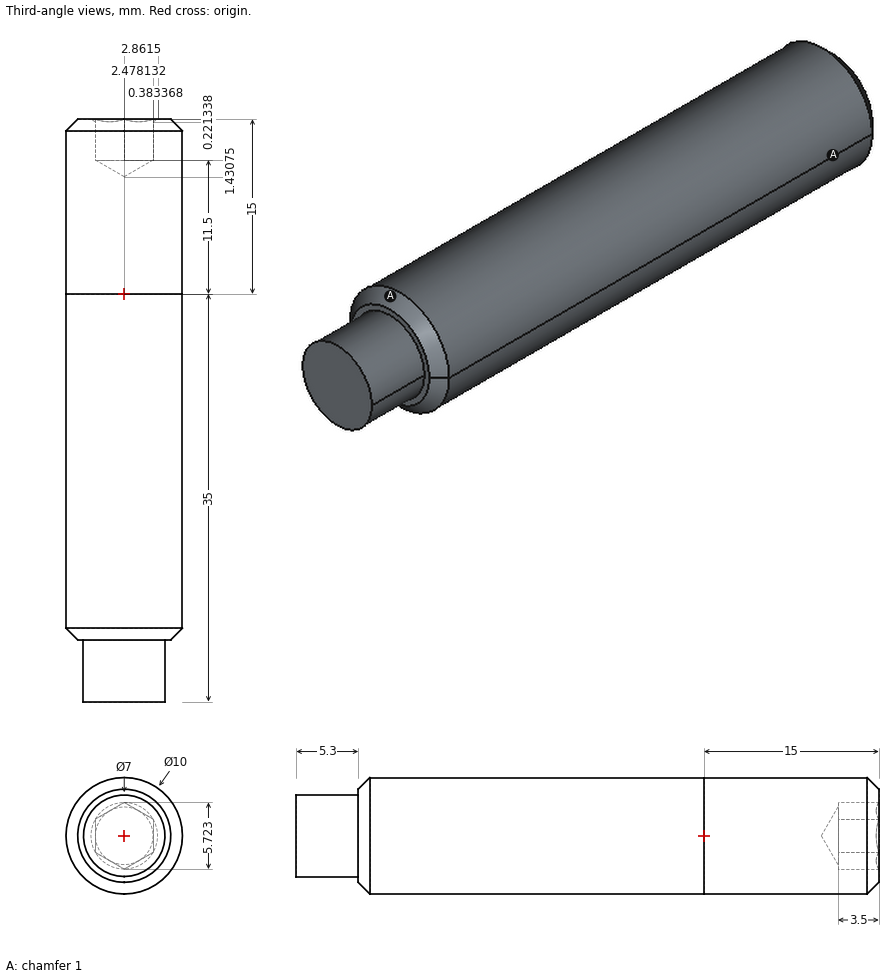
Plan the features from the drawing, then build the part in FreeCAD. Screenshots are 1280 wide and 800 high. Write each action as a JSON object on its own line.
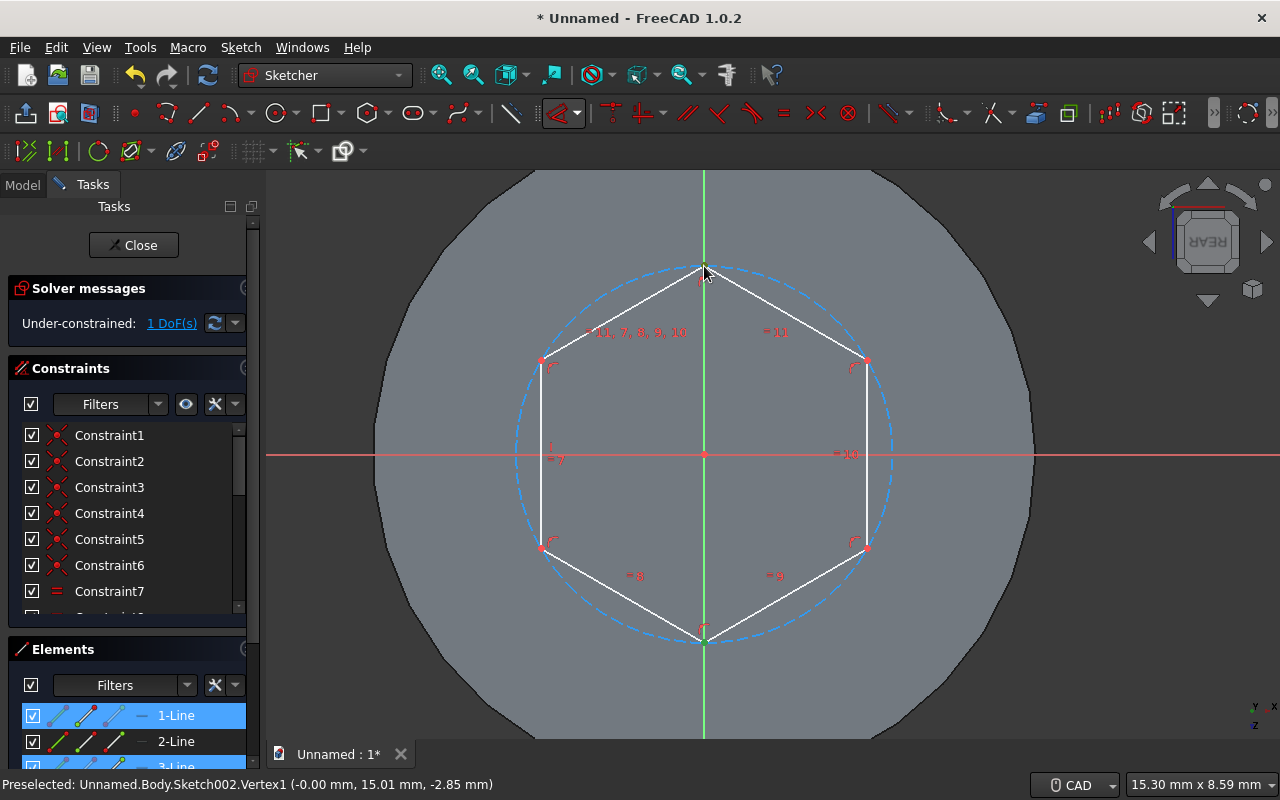
{"action": "left_click", "coordinate": [580, 114]}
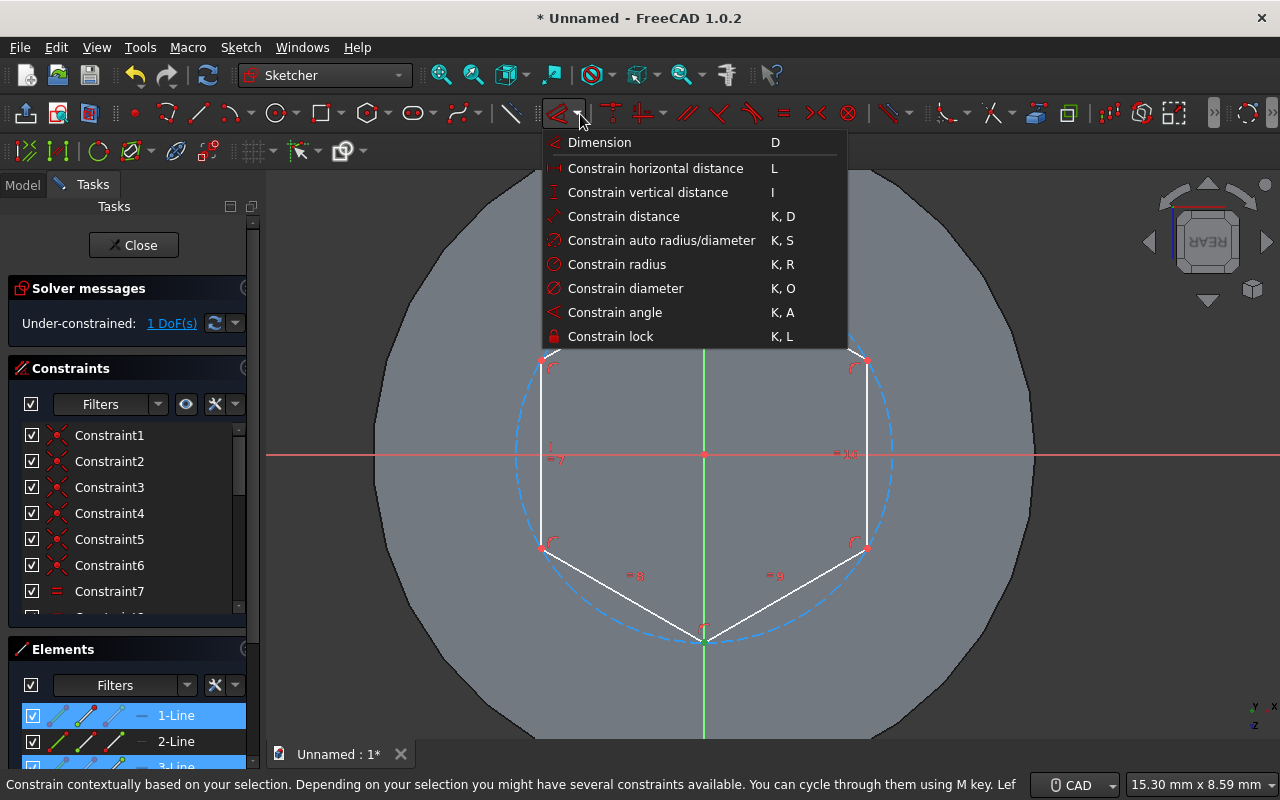
{"action": "left_click", "coordinate": [695, 192]}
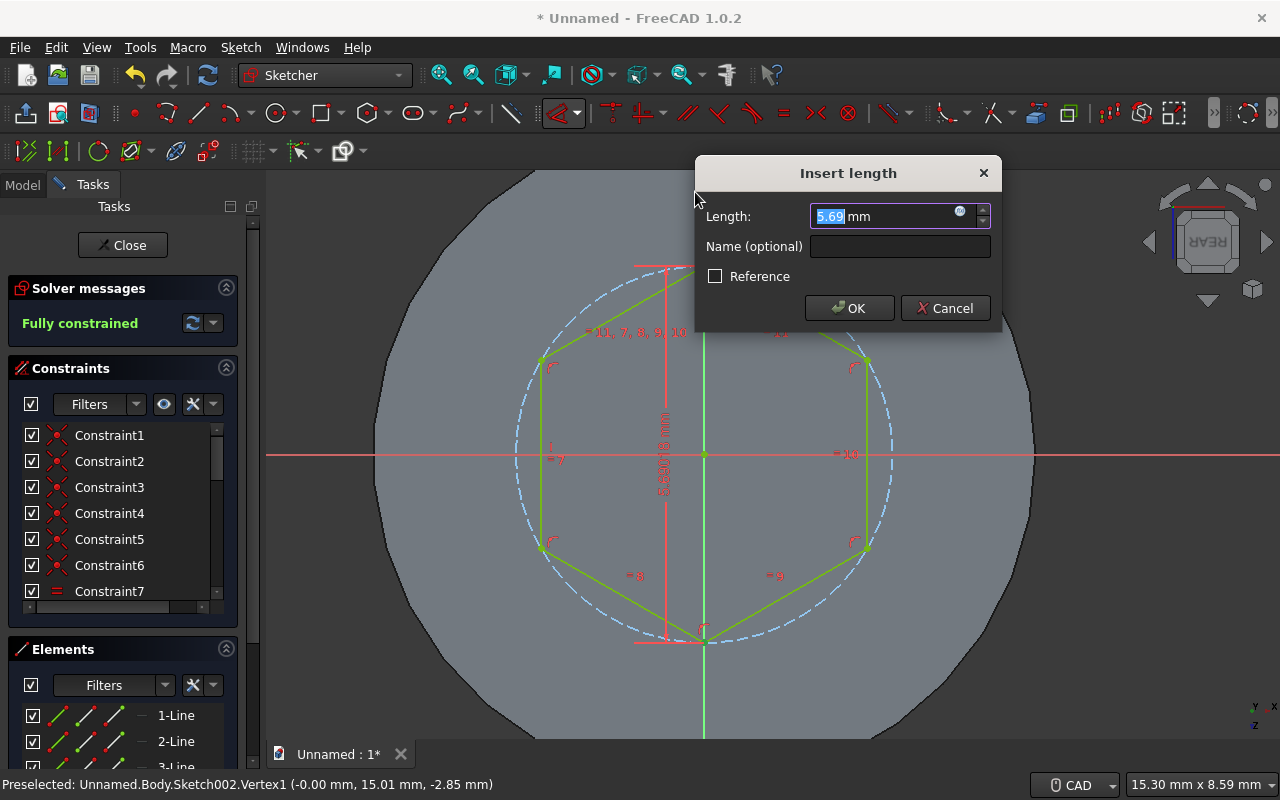
{"action": "type", "text": "5.723"}
{"action": "key", "text": "Return"}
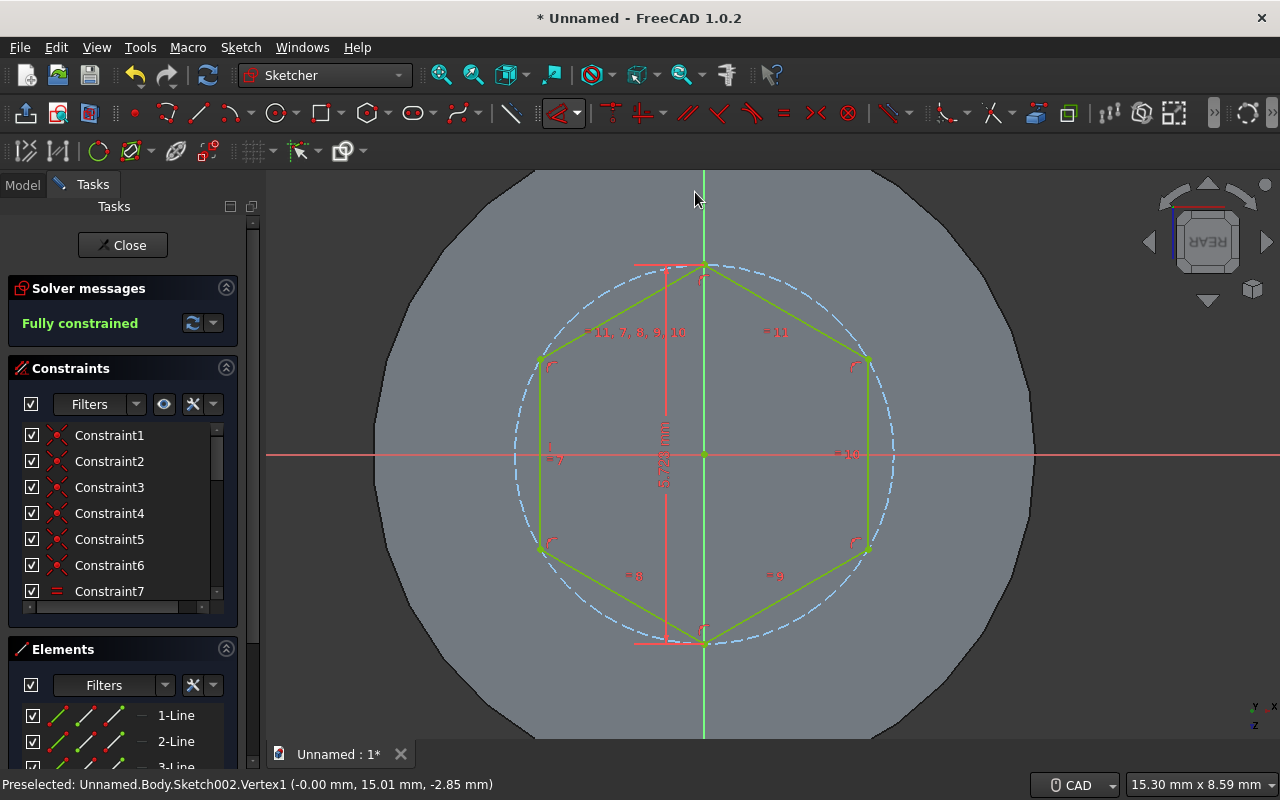
{"action": "left_click", "coordinate": [123, 245]}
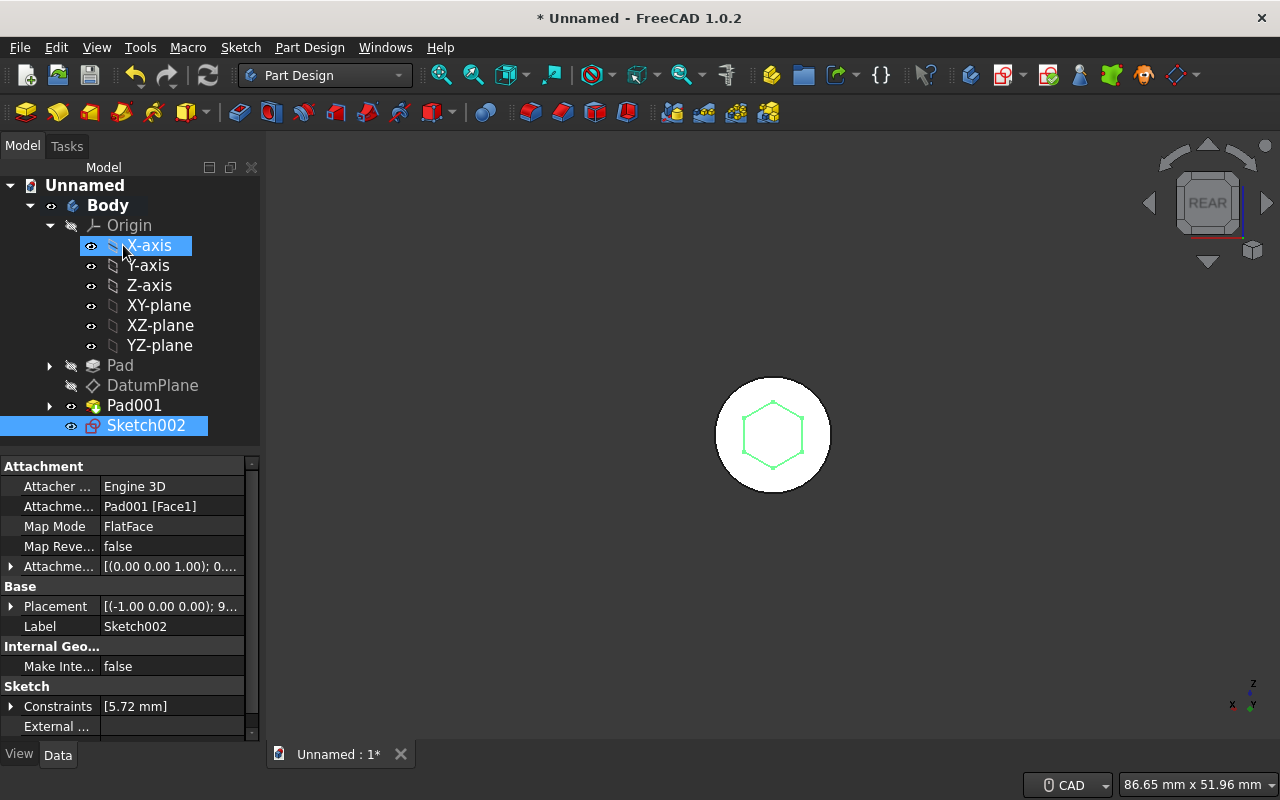
{"action": "left_click", "coordinate": [240, 112]}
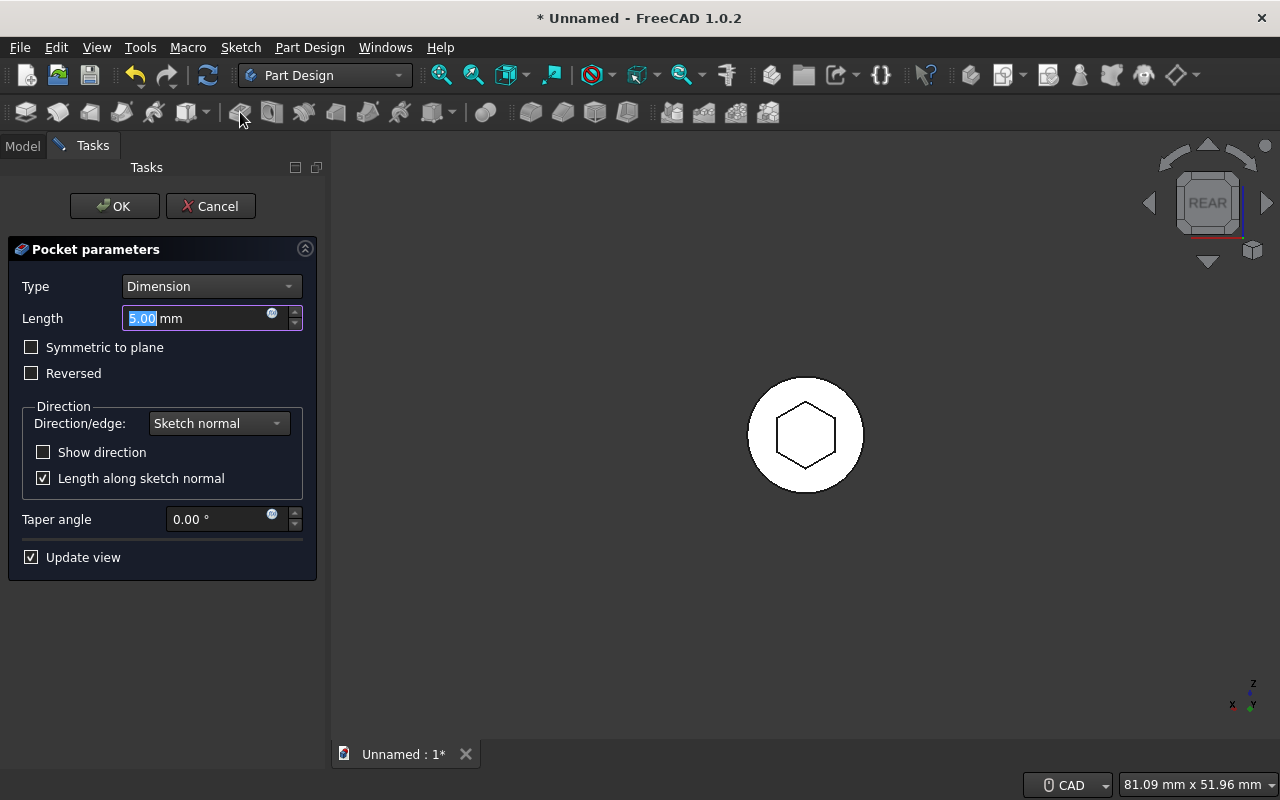
{"action": "type", "text": "3.5"}
{"action": "key", "text": "Tab"}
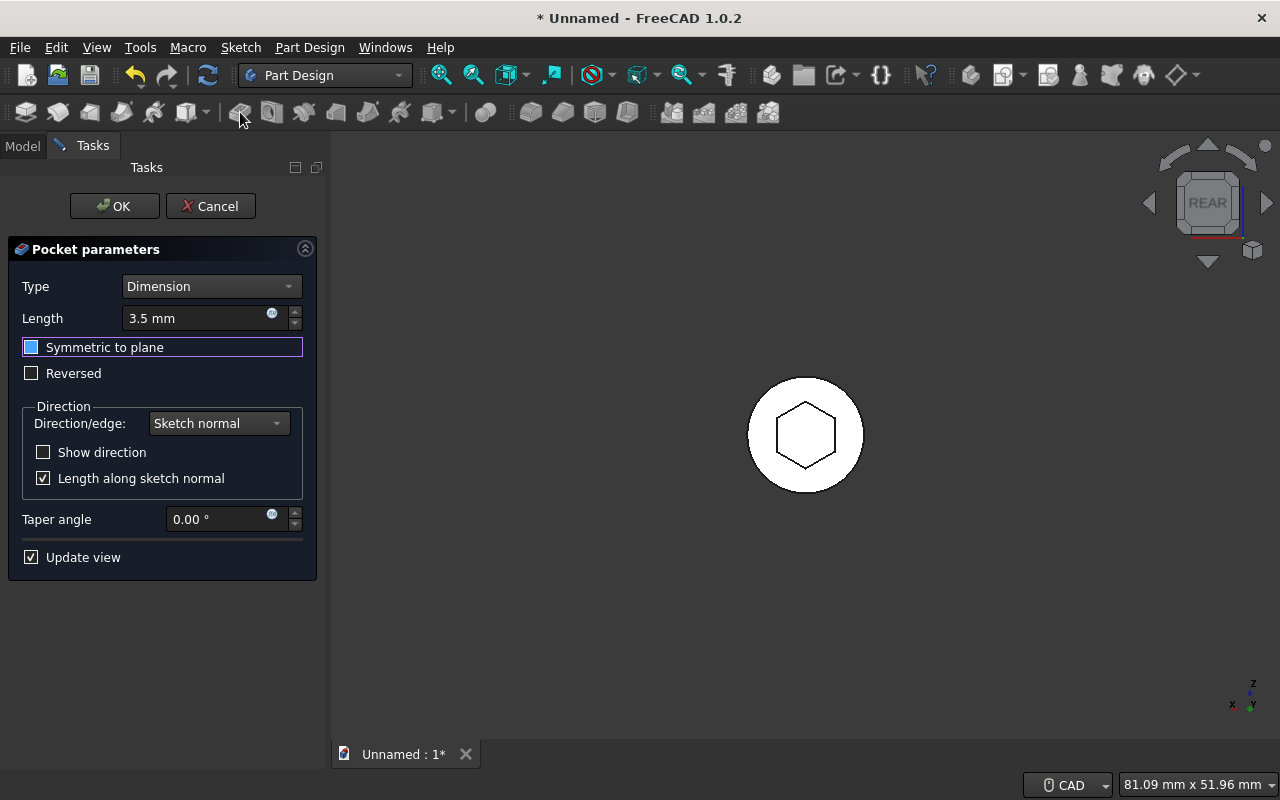
{"action": "left_click", "coordinate": [115, 206]}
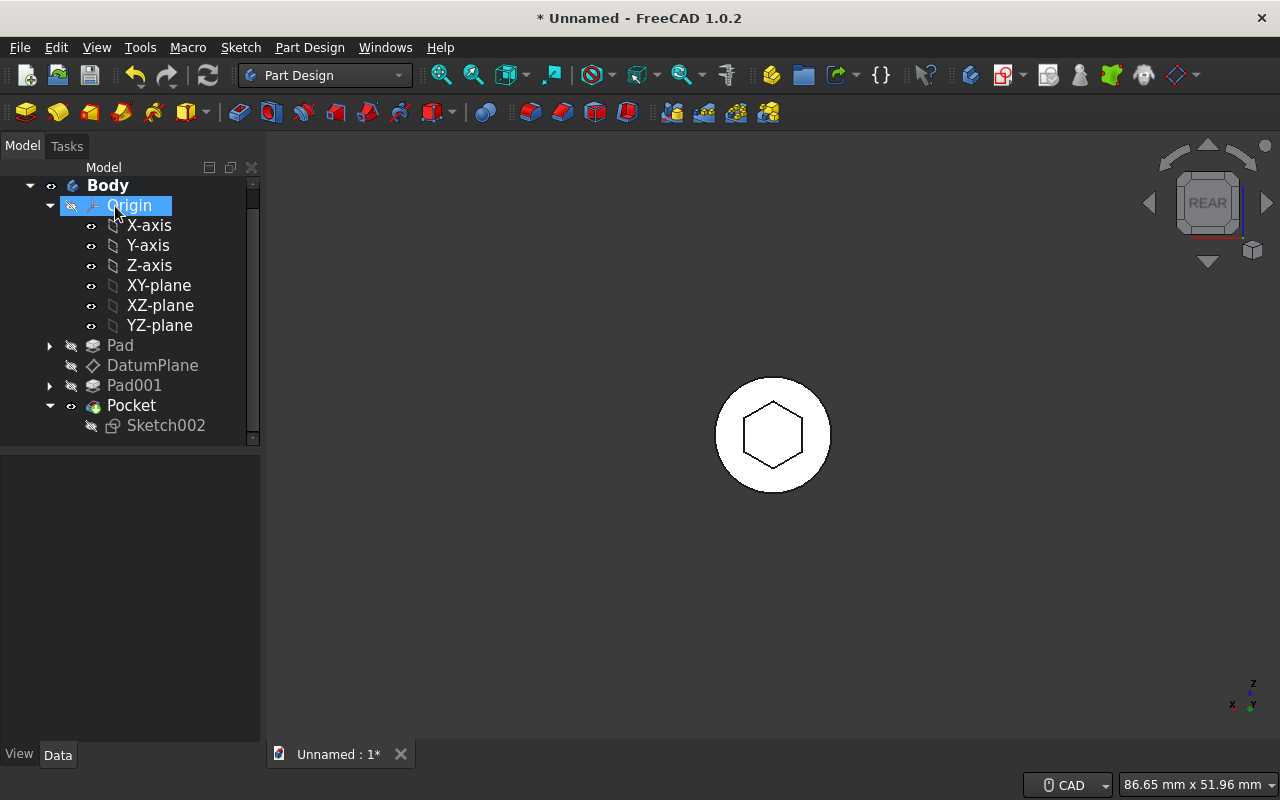
{"action": "left_click", "coordinate": [442, 76]}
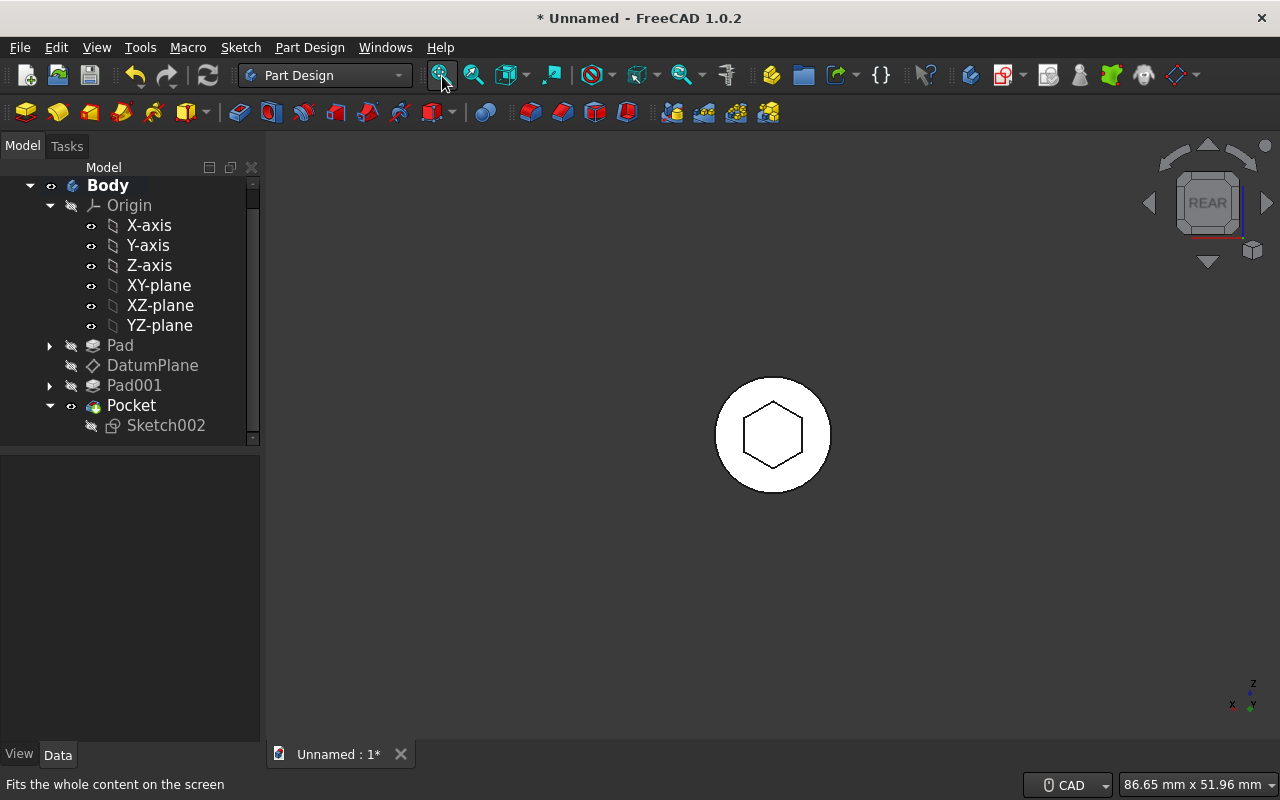
{"action": "left_click", "coordinate": [1004, 76]}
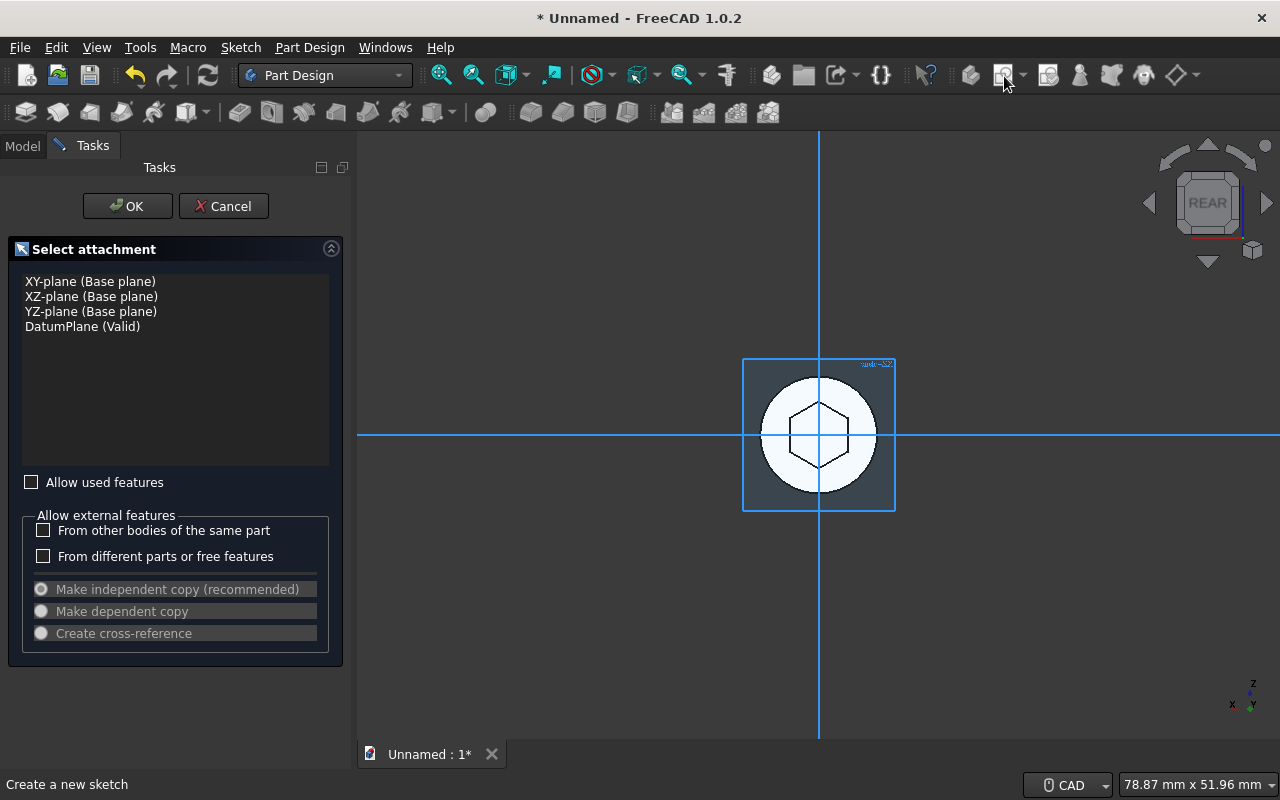
{"action": "left_click", "coordinate": [82, 282]}